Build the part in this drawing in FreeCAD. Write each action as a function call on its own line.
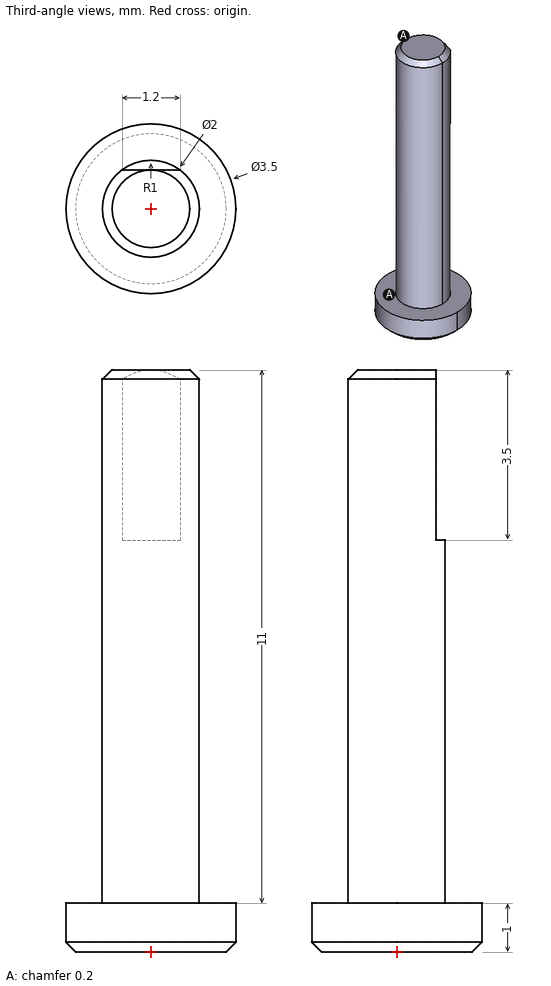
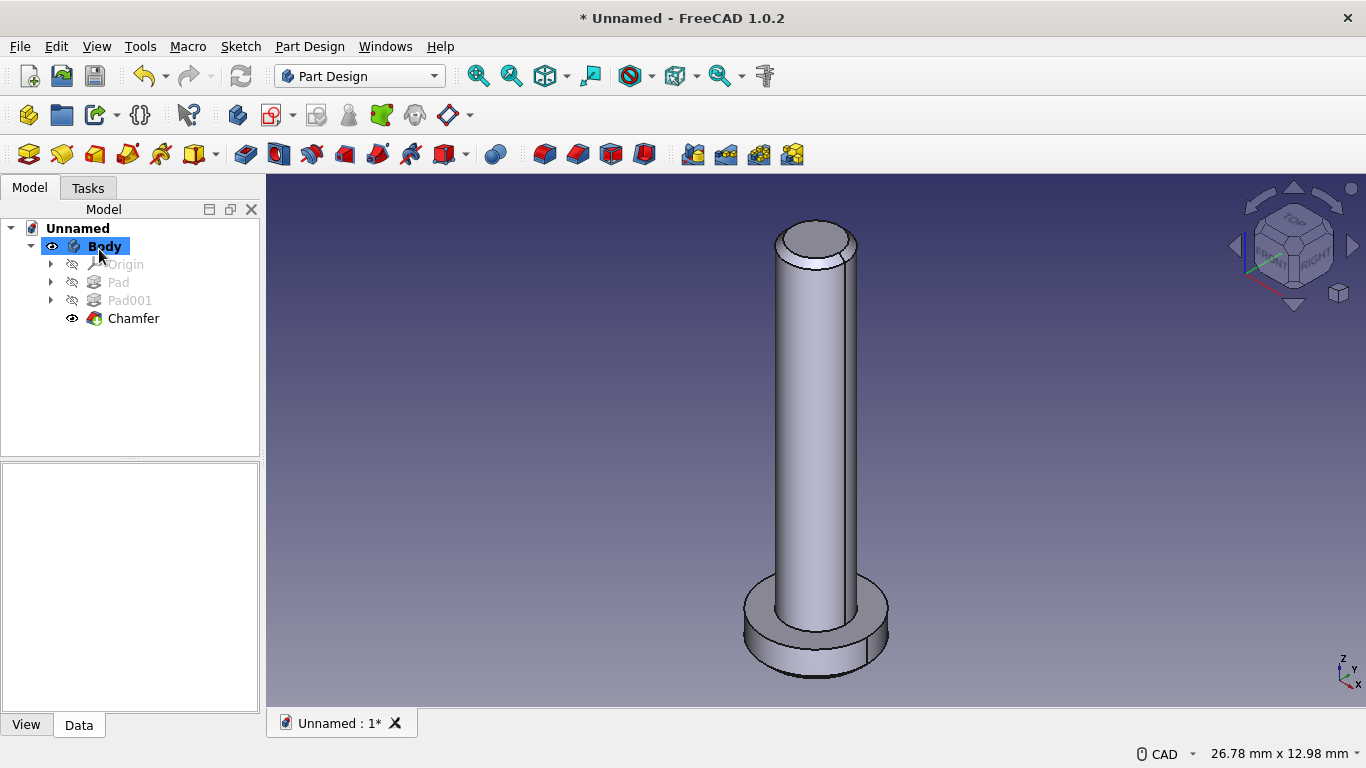
click(51, 264)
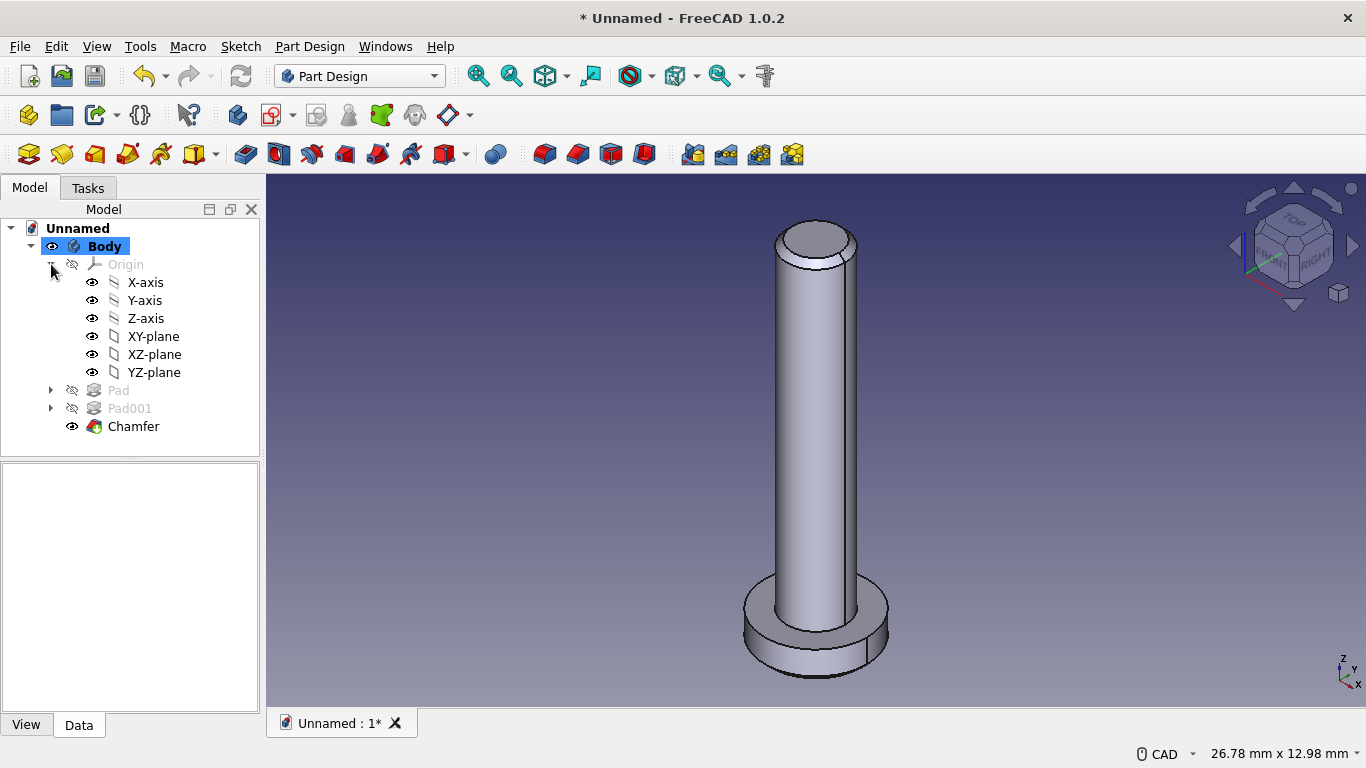
click(137, 336)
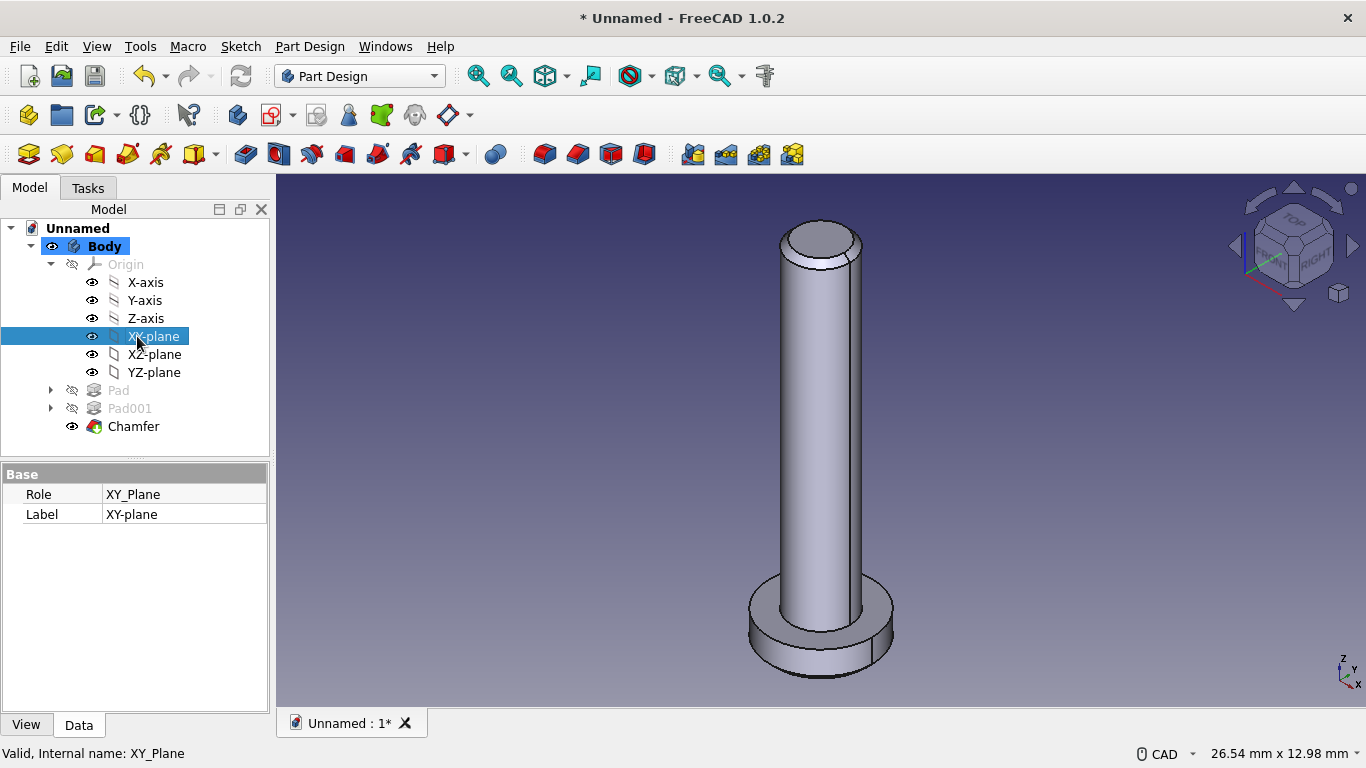
click(448, 116)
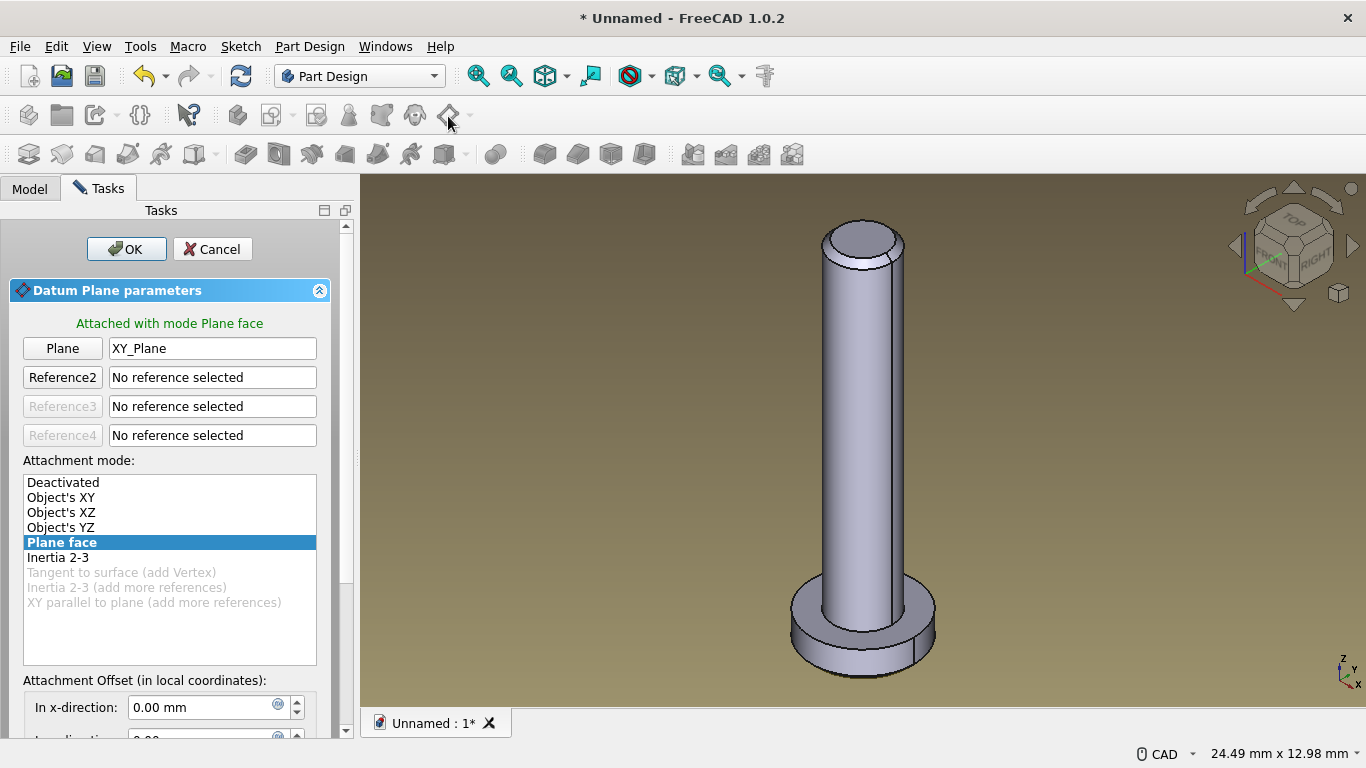
scroll(346, 479, down, 2)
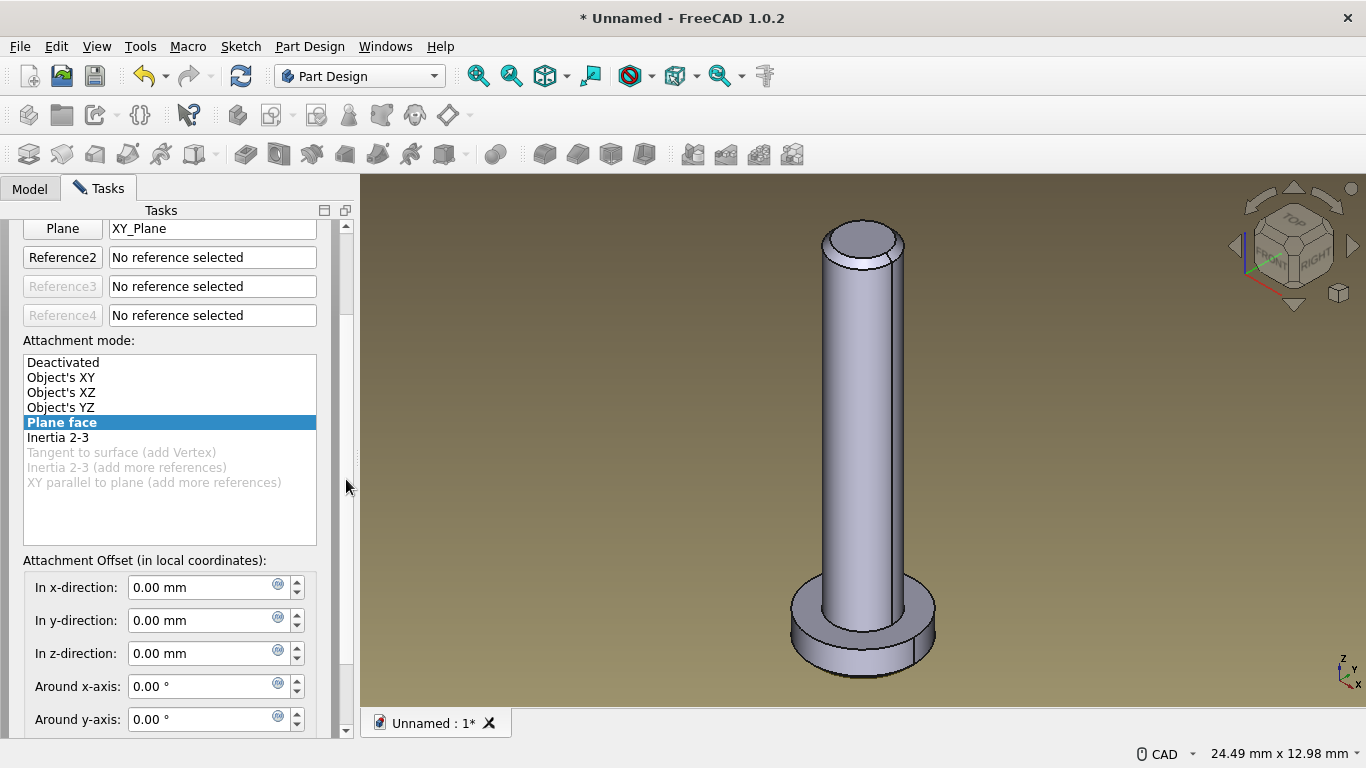
triple_click(210, 654)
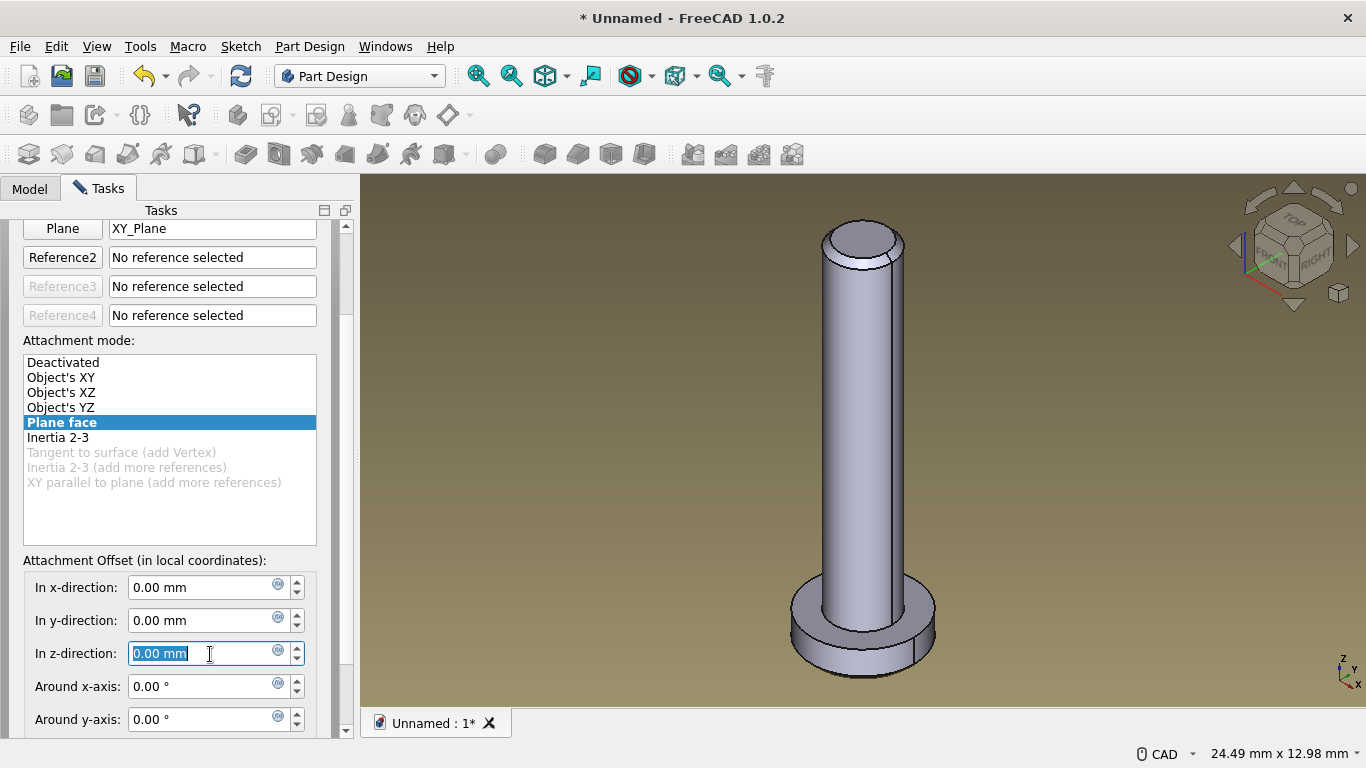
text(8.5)
key(Tab)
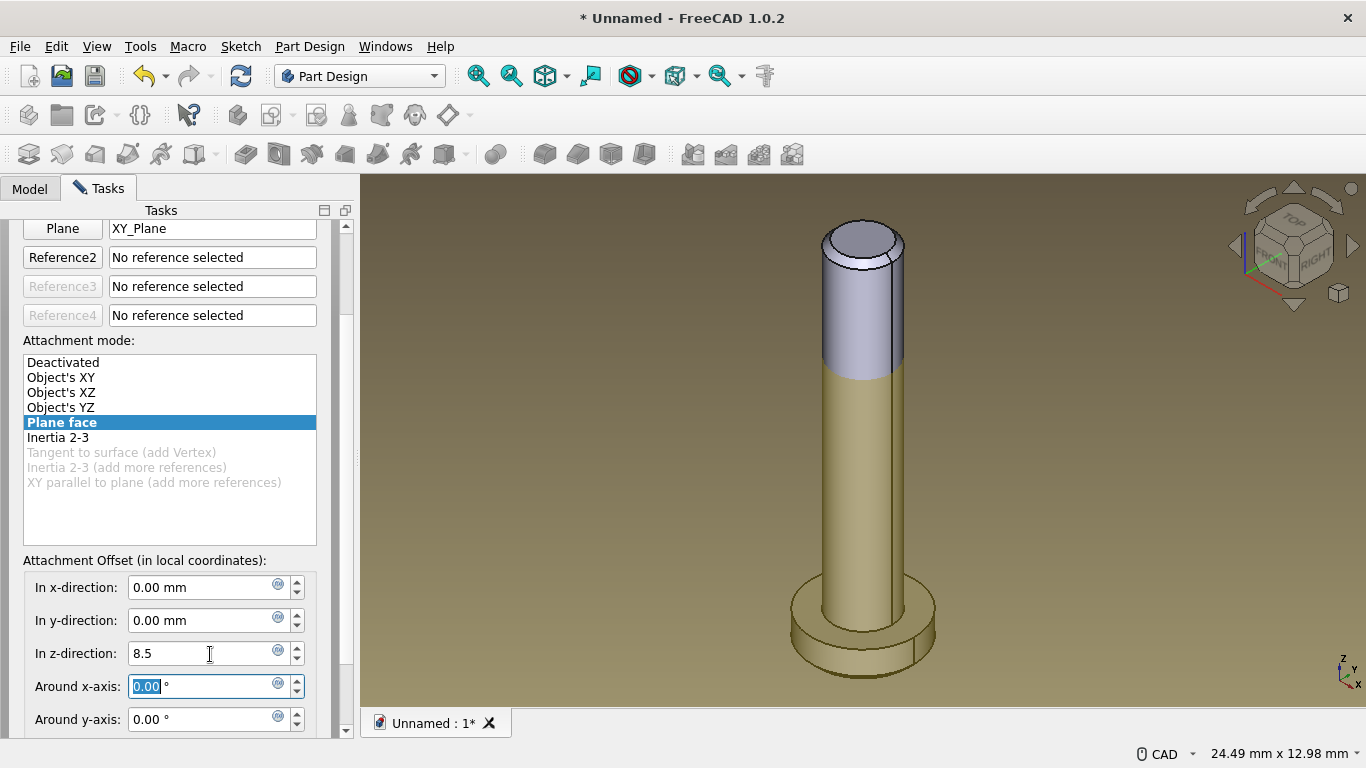
scroll(346, 479, up, 3)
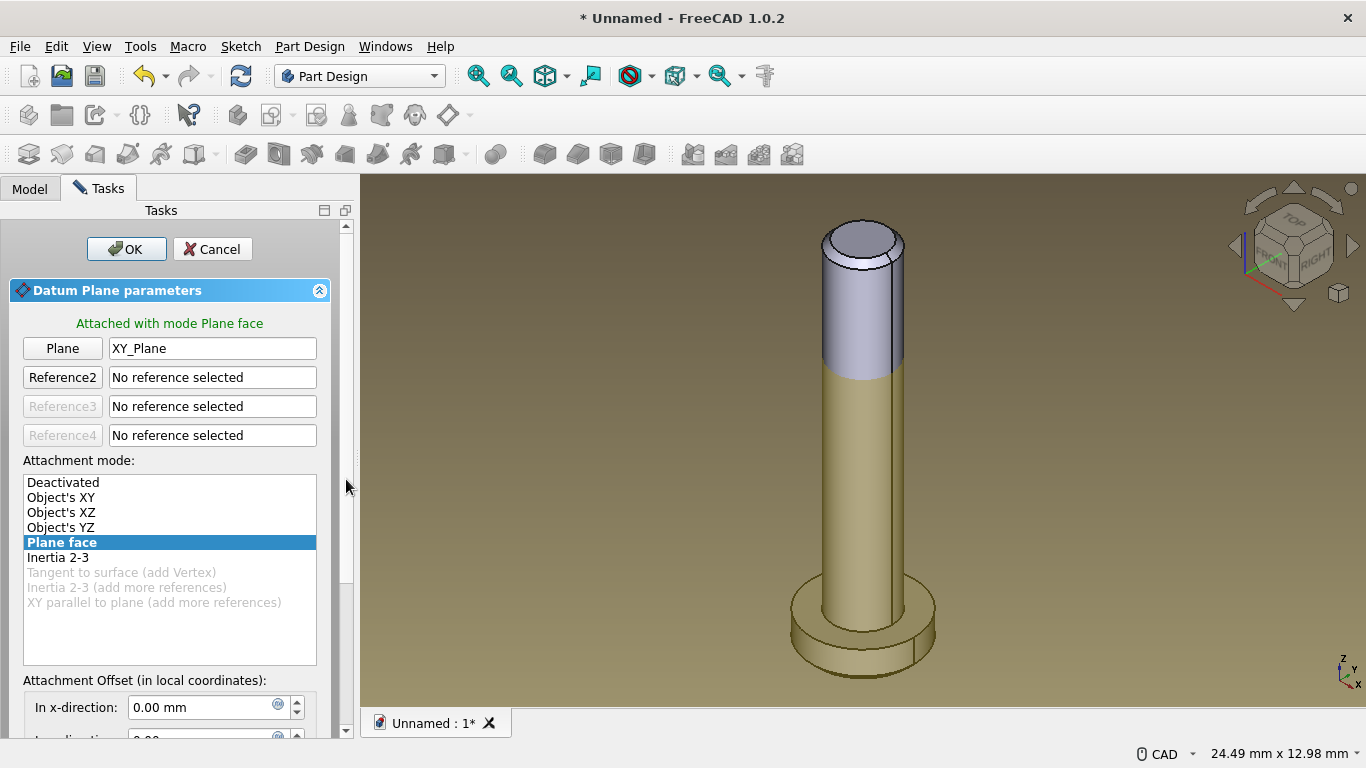
click(127, 249)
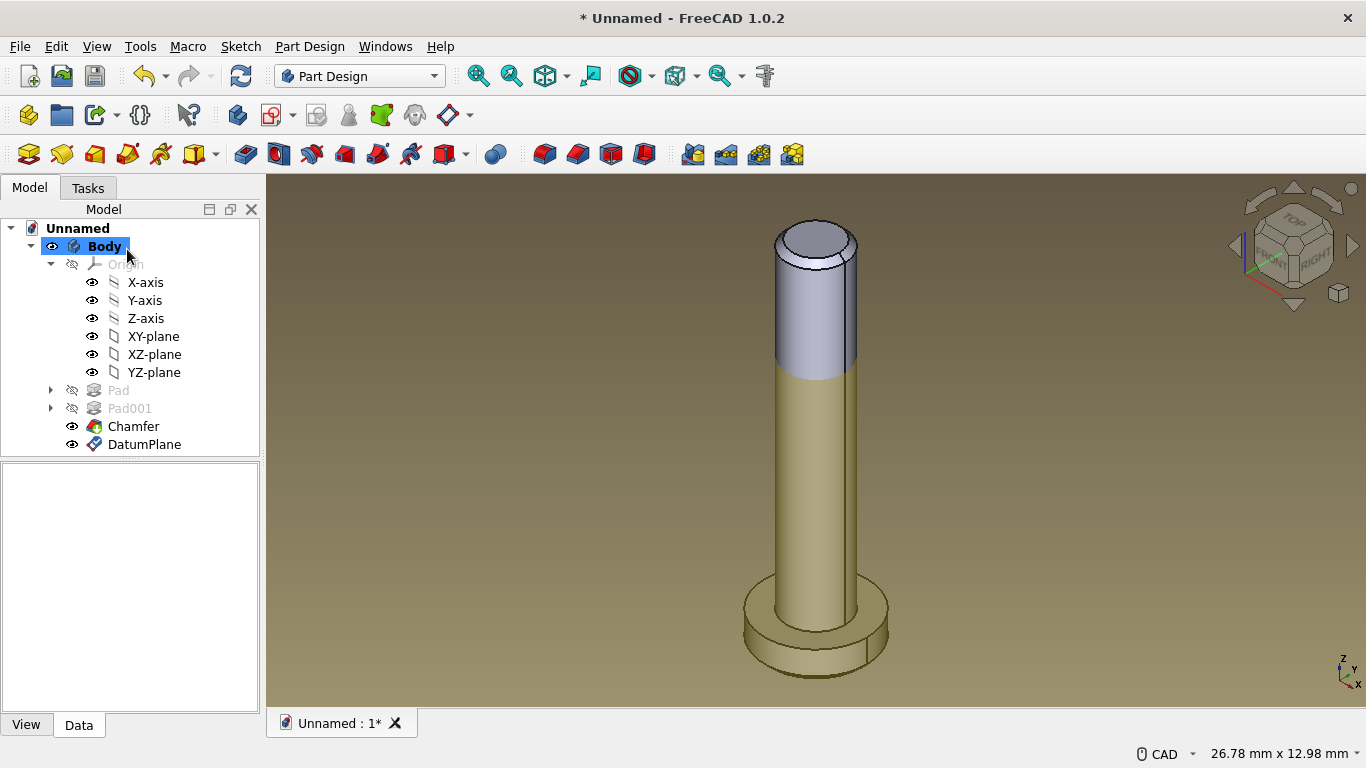
click(117, 444)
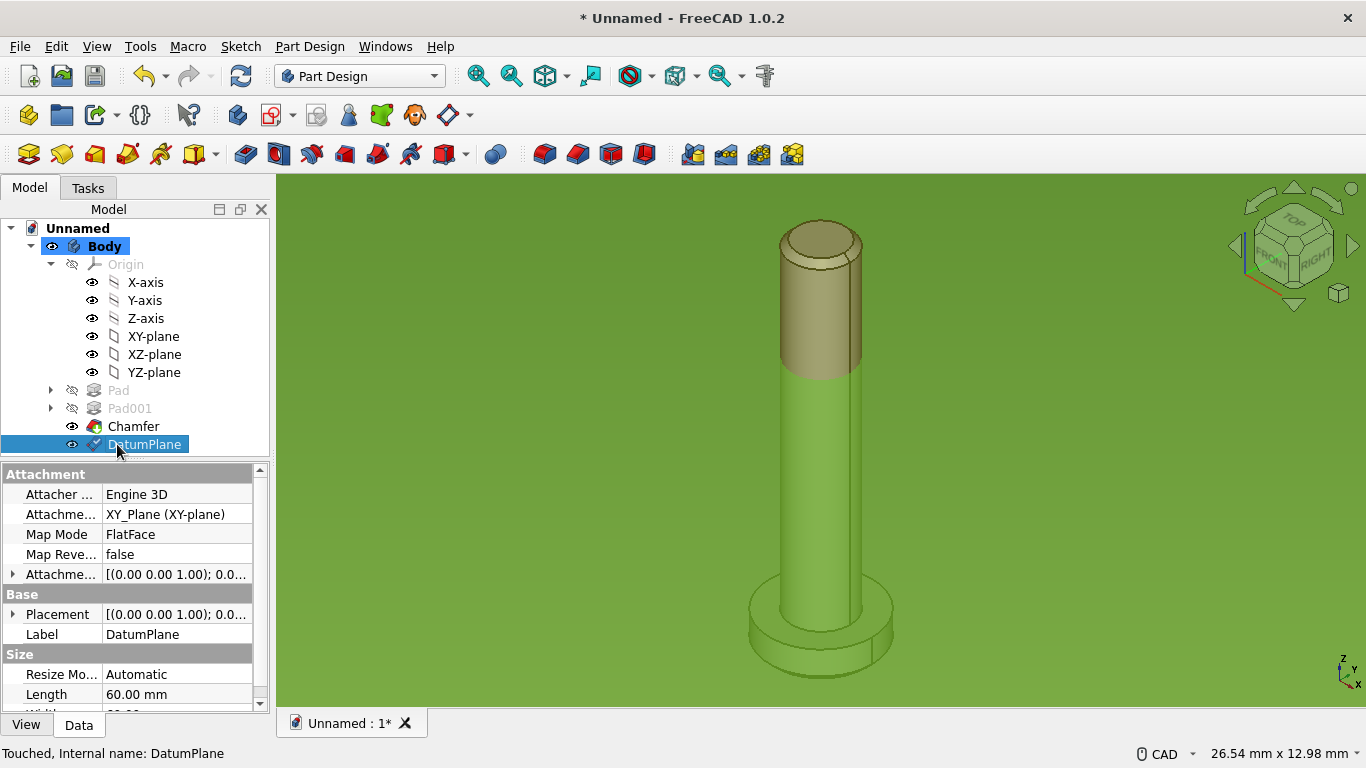
click(270, 116)